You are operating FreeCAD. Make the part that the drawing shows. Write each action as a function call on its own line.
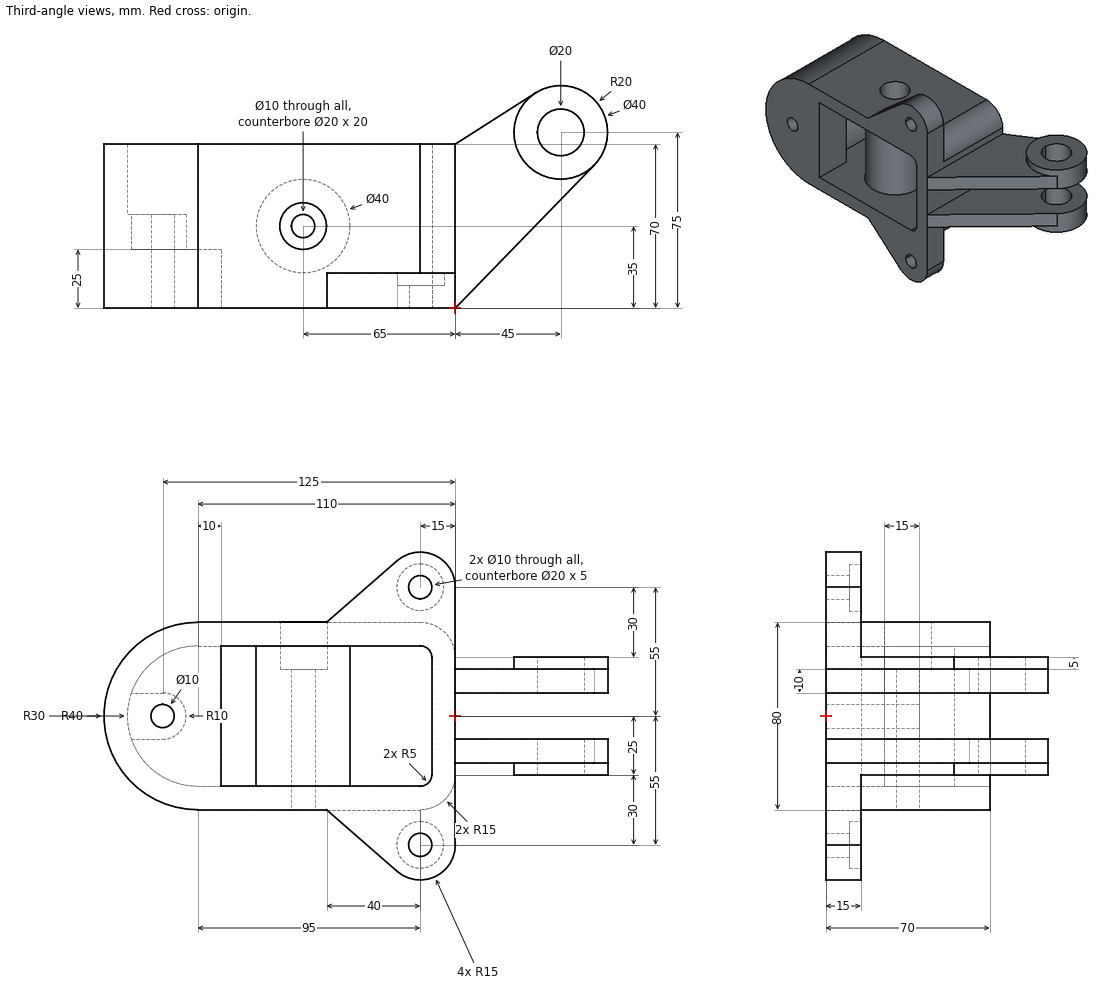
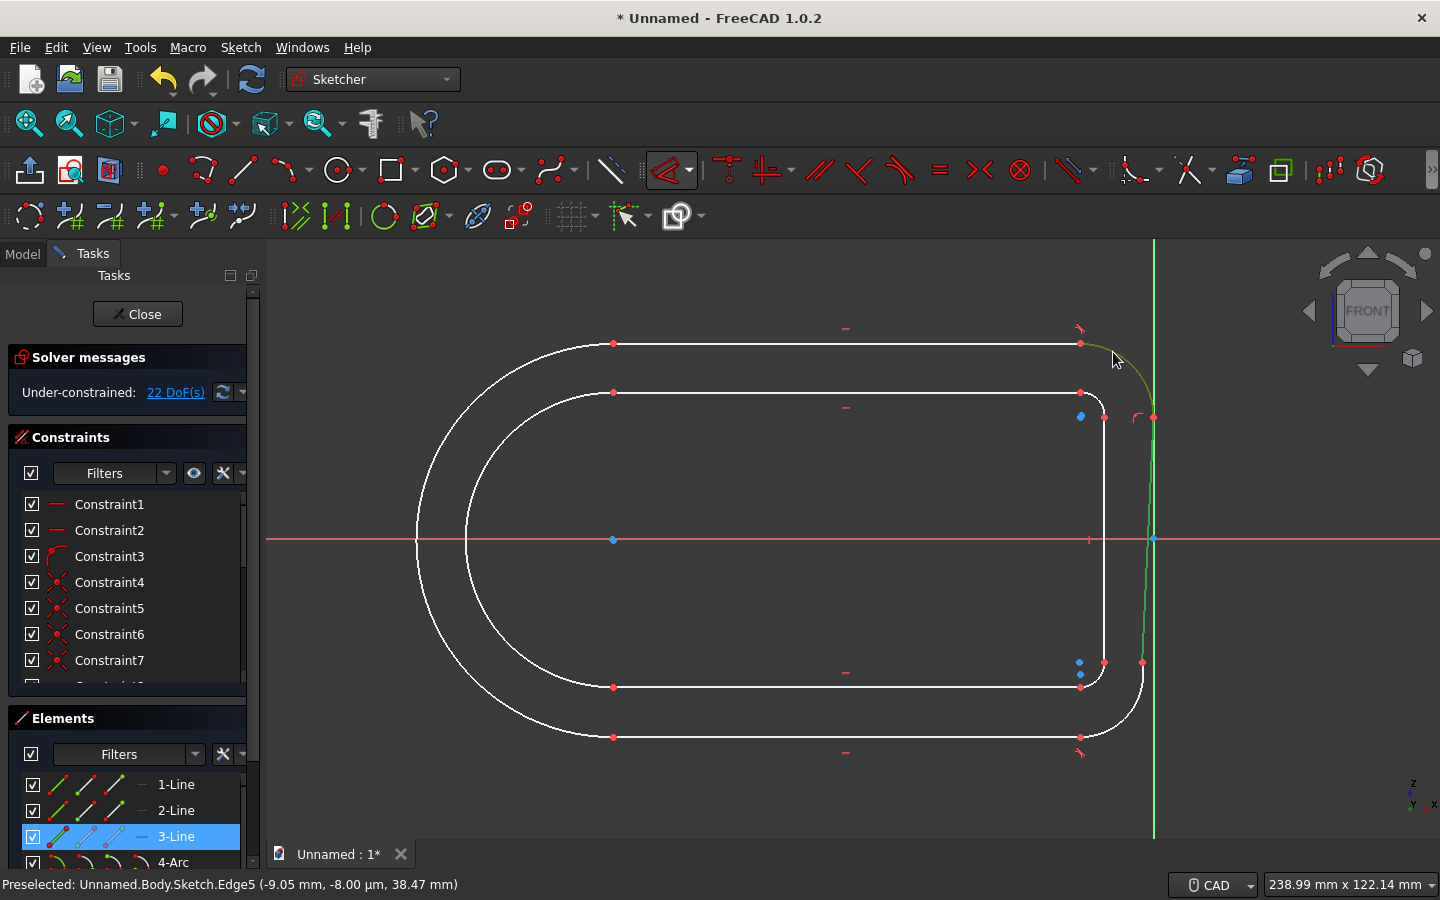
key(t)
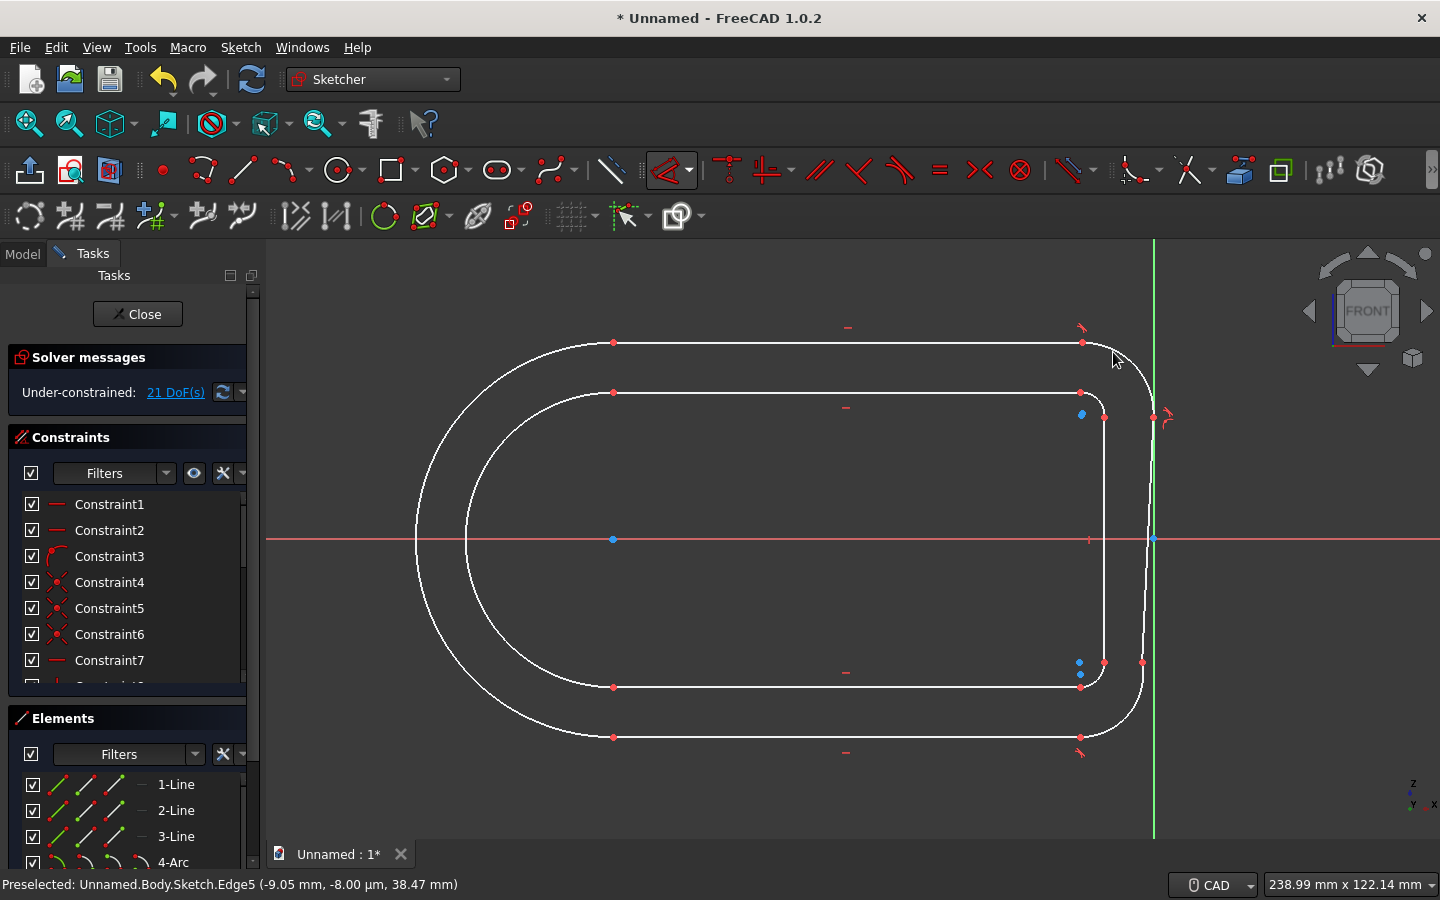
click(1150, 491)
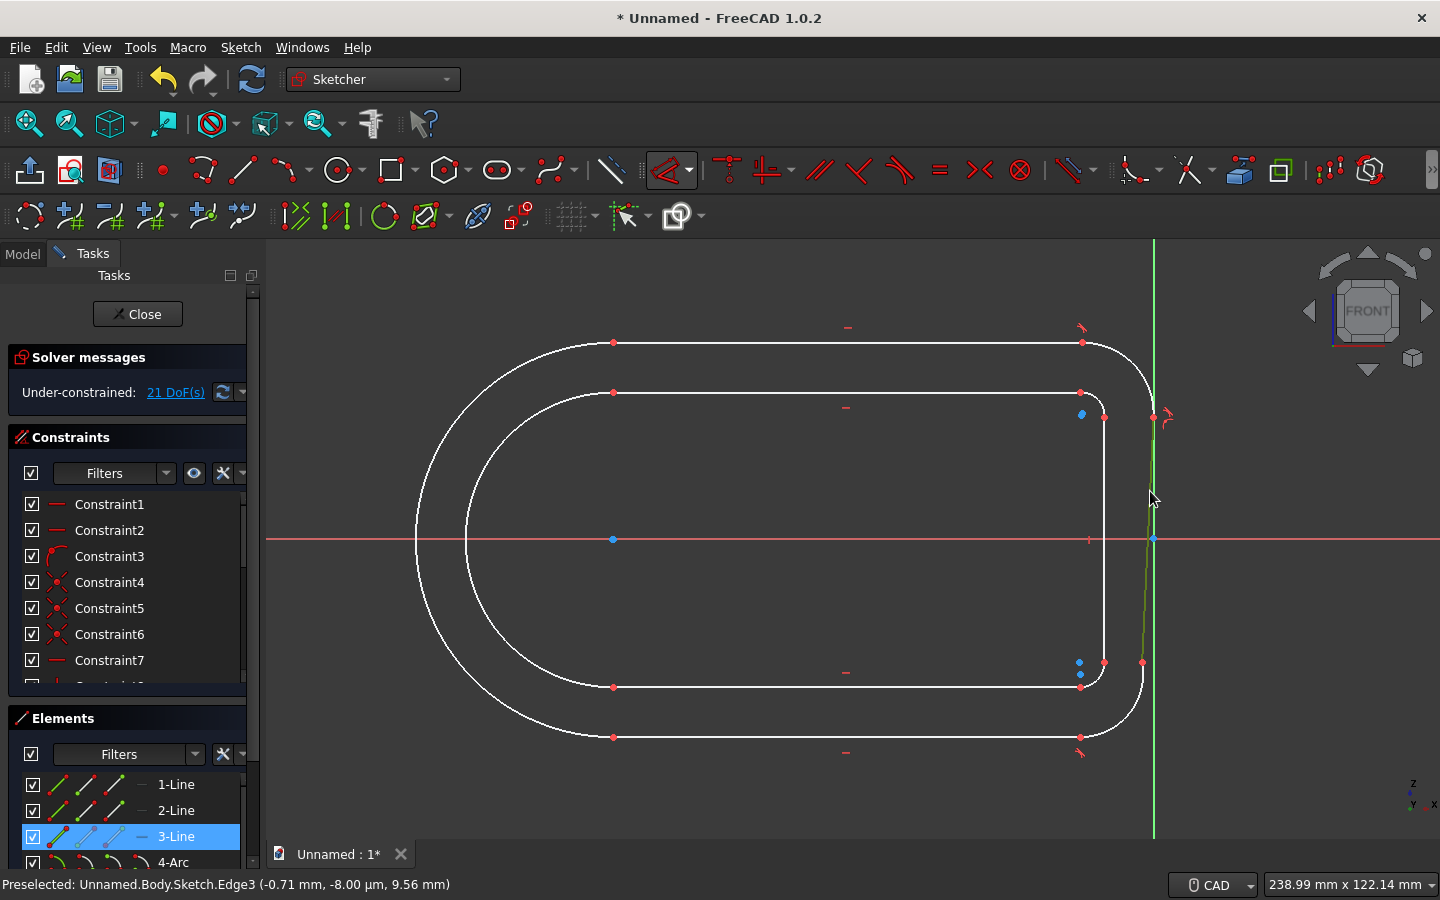
click(1112, 729)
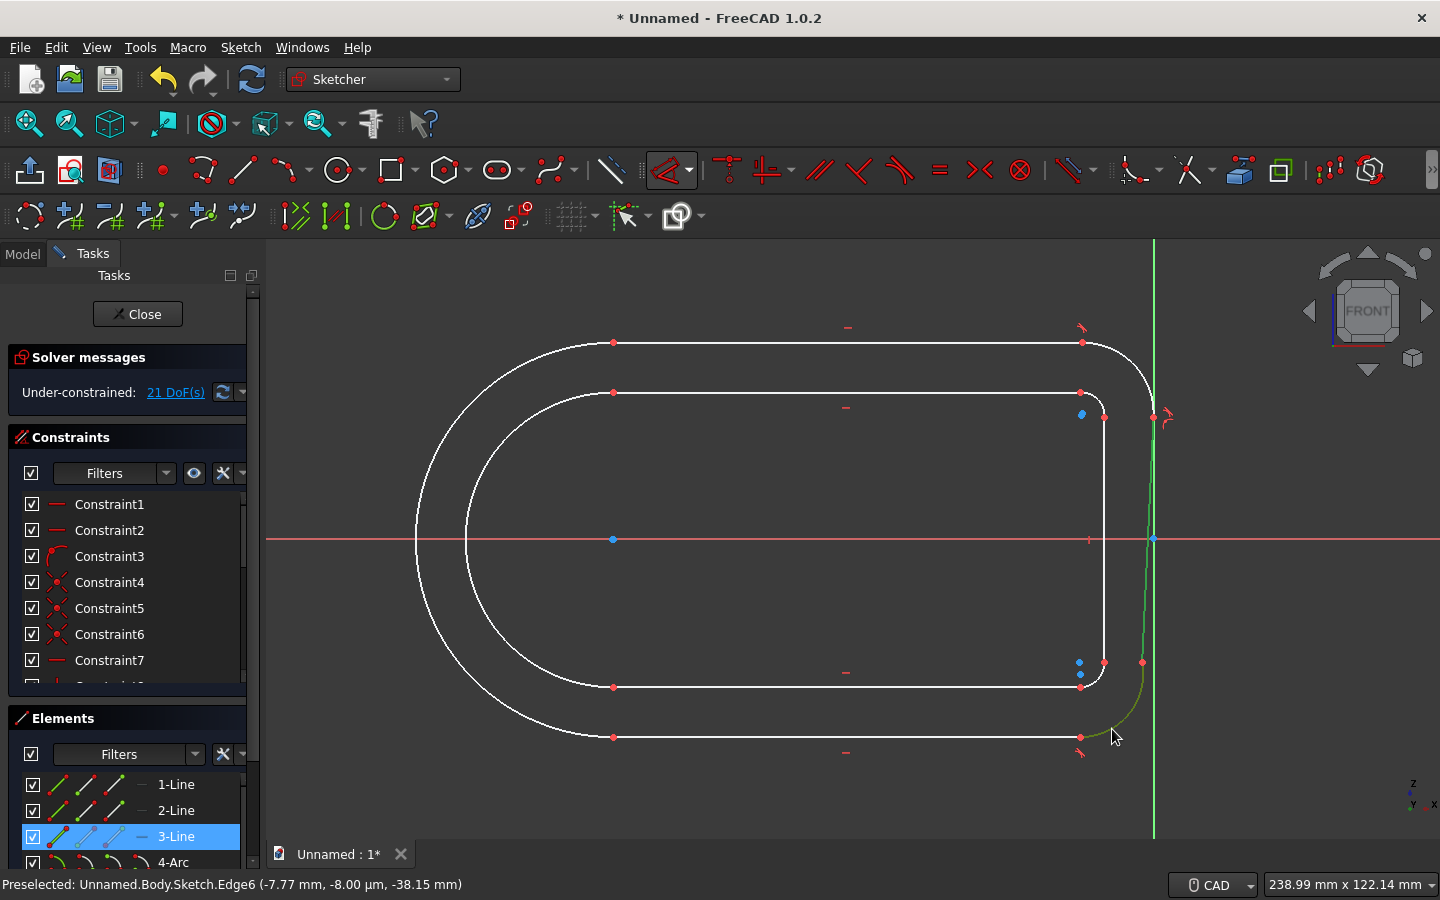
click(900, 170)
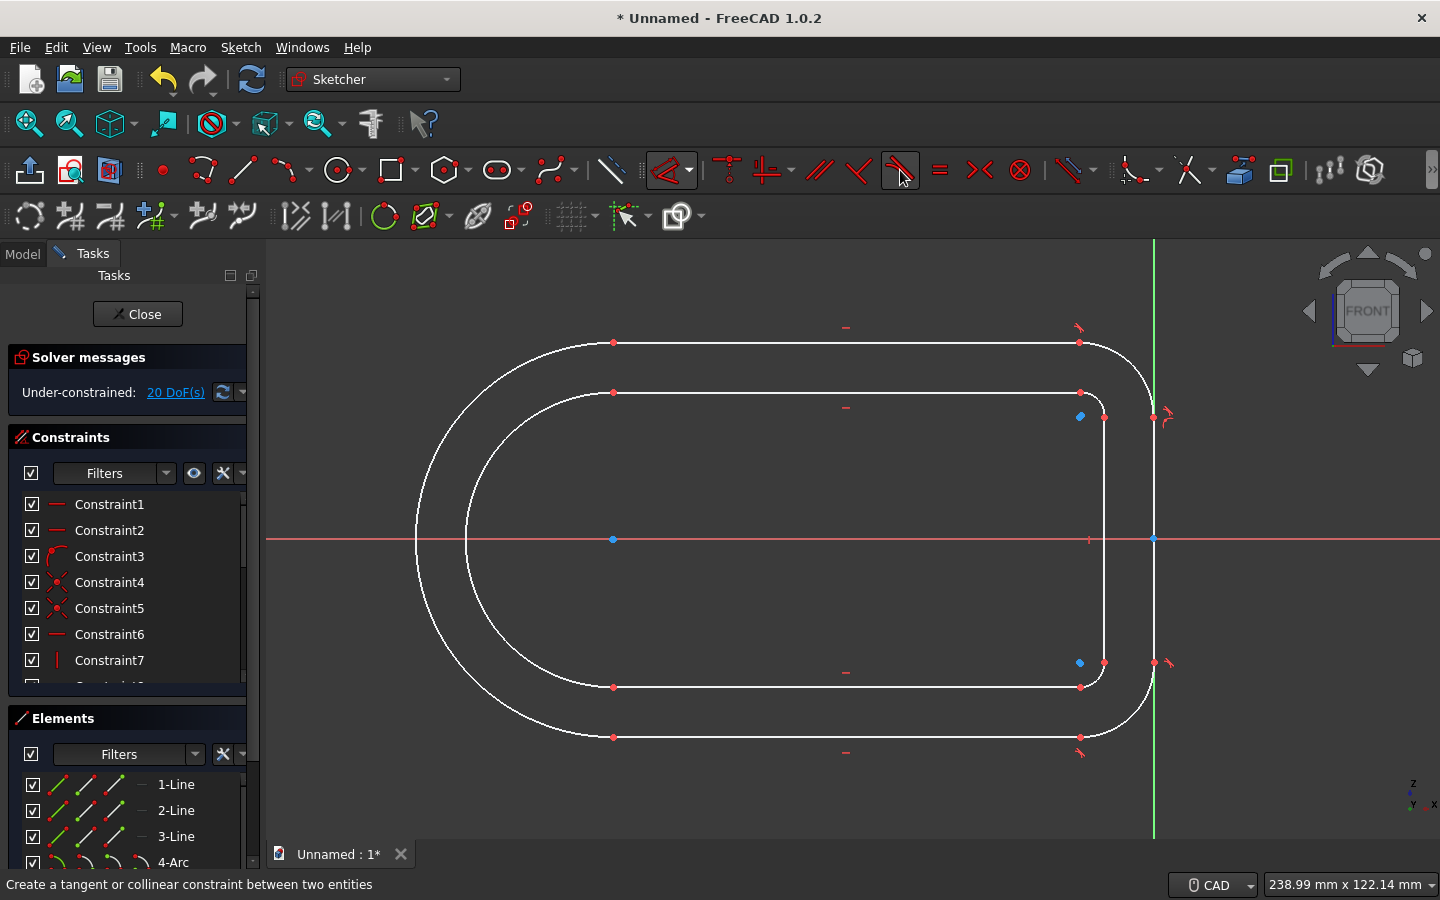
click(754, 687)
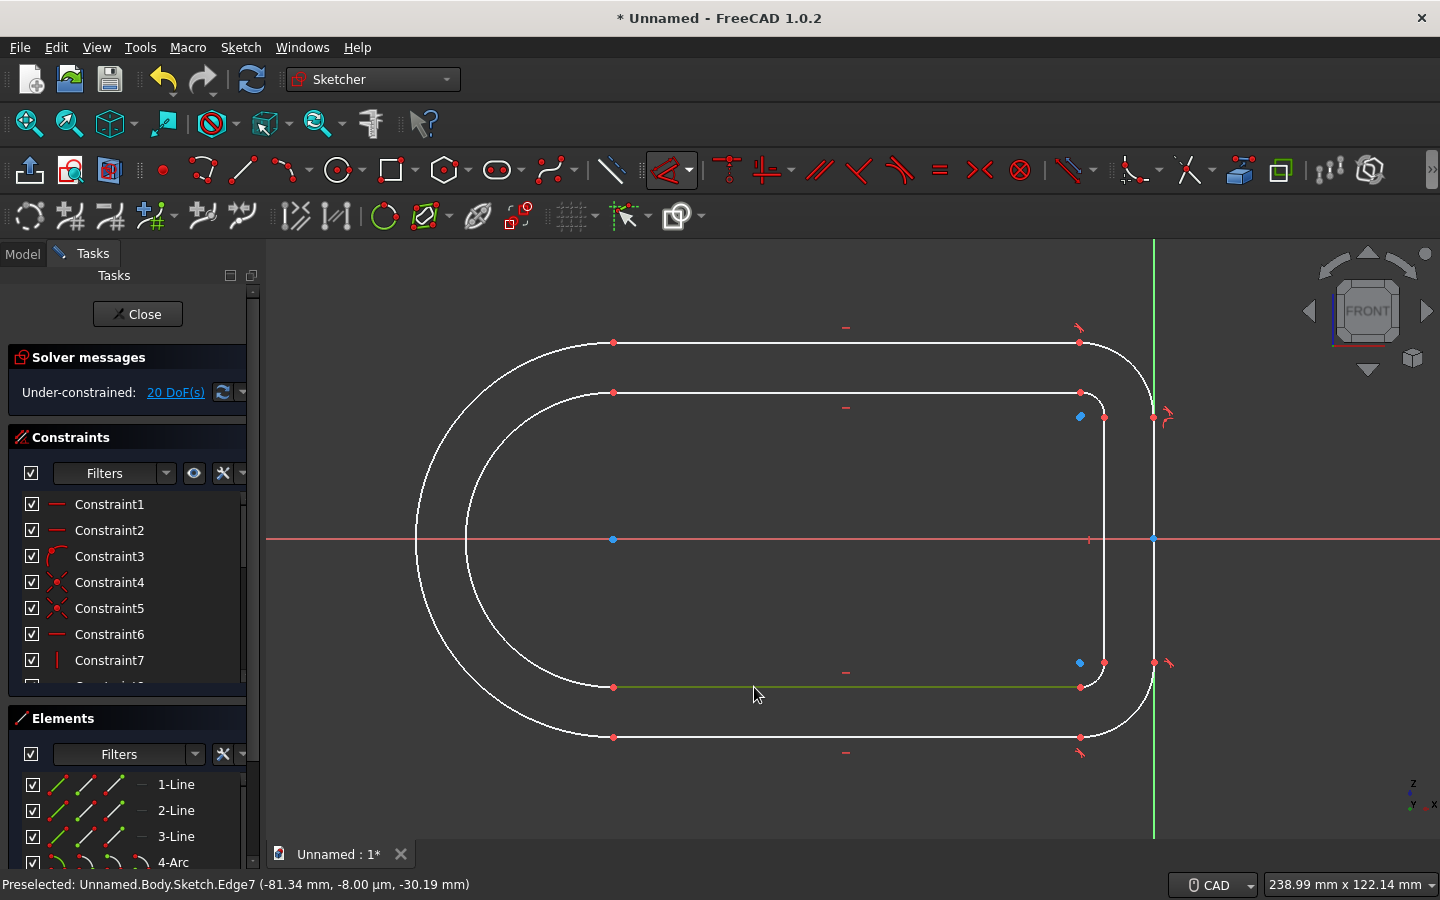
click(1091, 685)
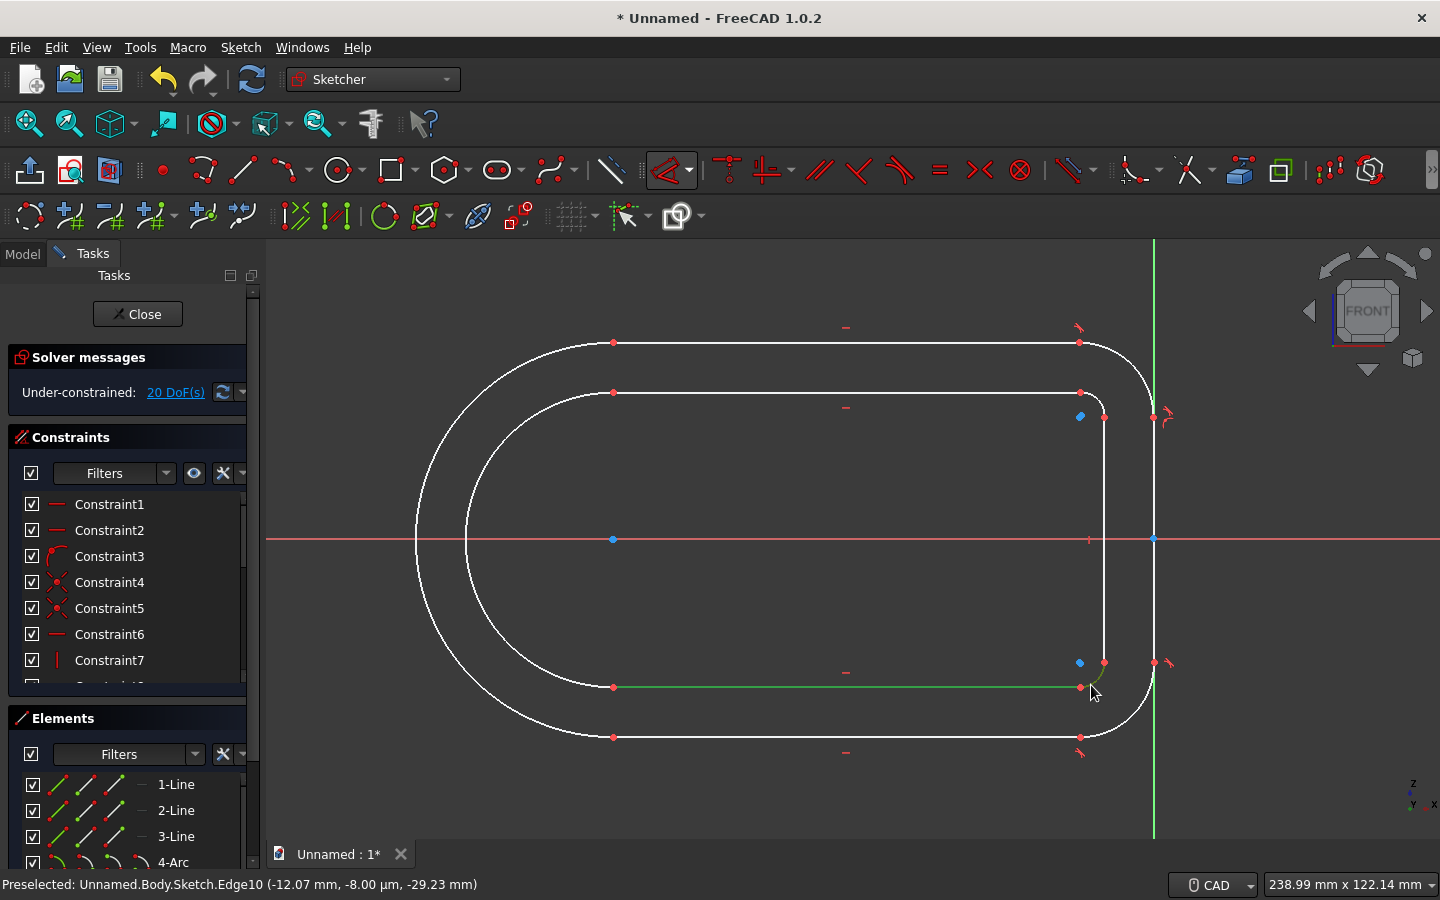
key(t)